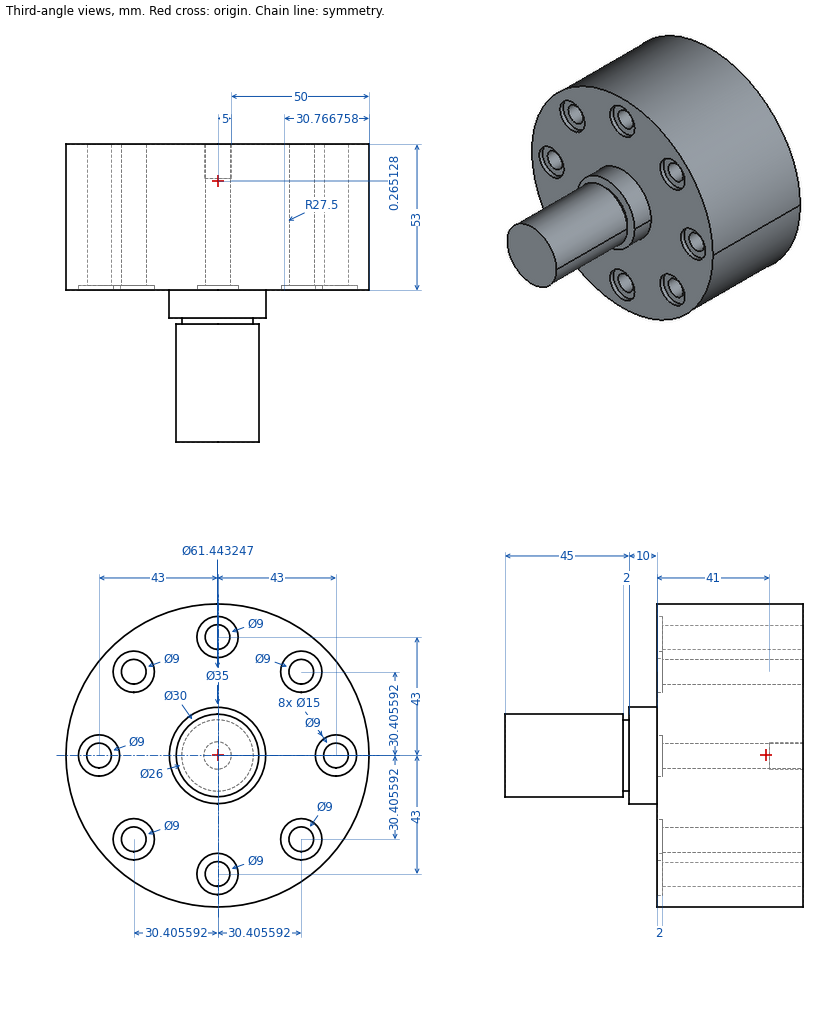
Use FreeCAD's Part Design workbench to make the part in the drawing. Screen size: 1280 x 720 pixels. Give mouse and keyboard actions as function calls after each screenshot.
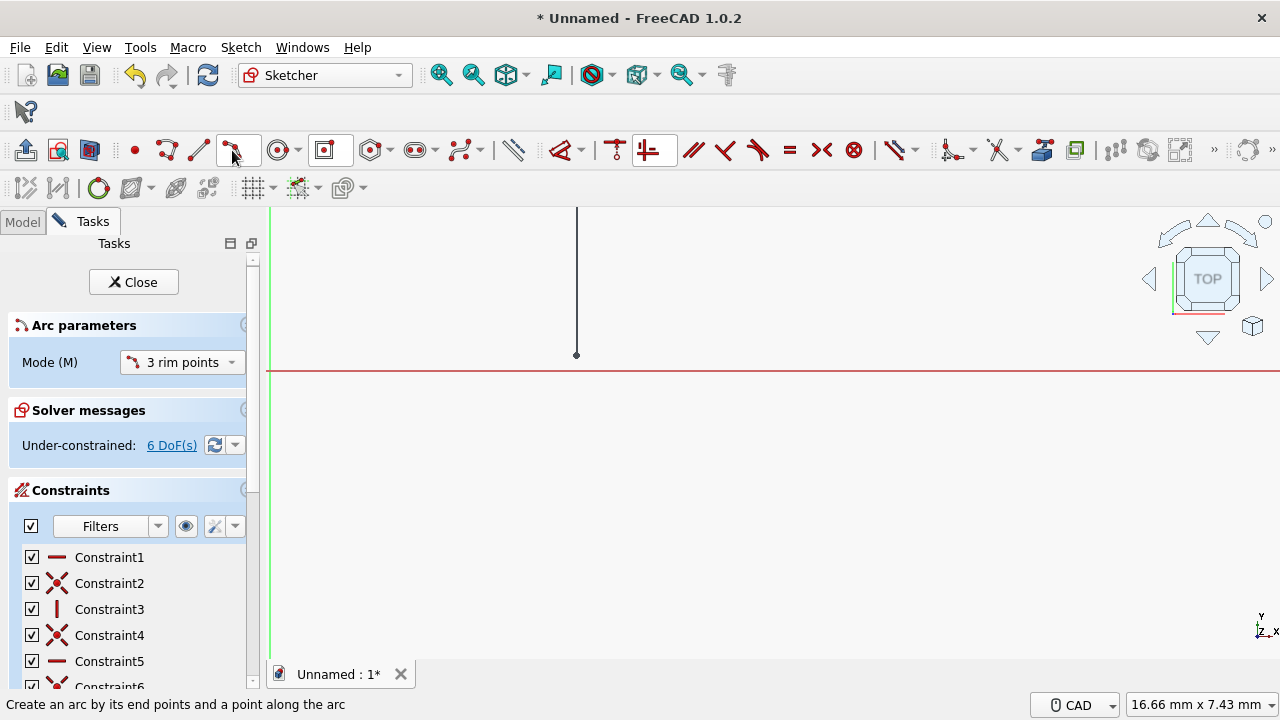
click(577, 356)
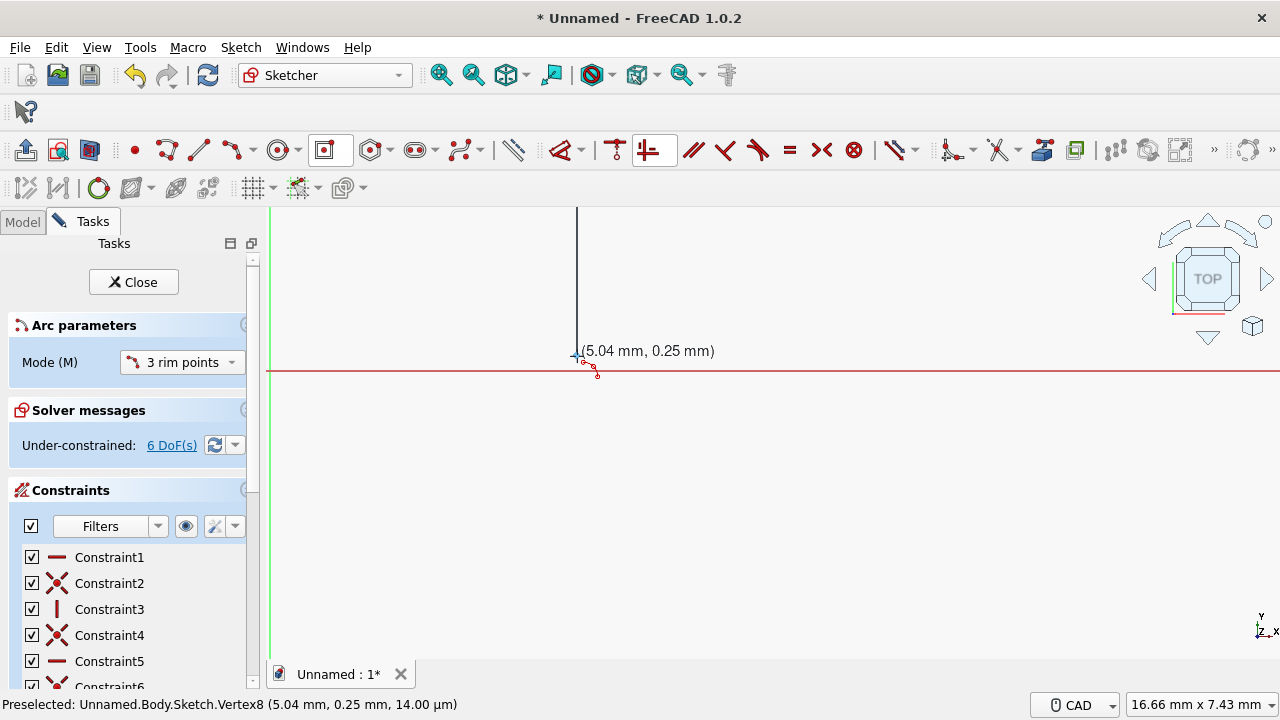
scroll(581, 359, down, 12)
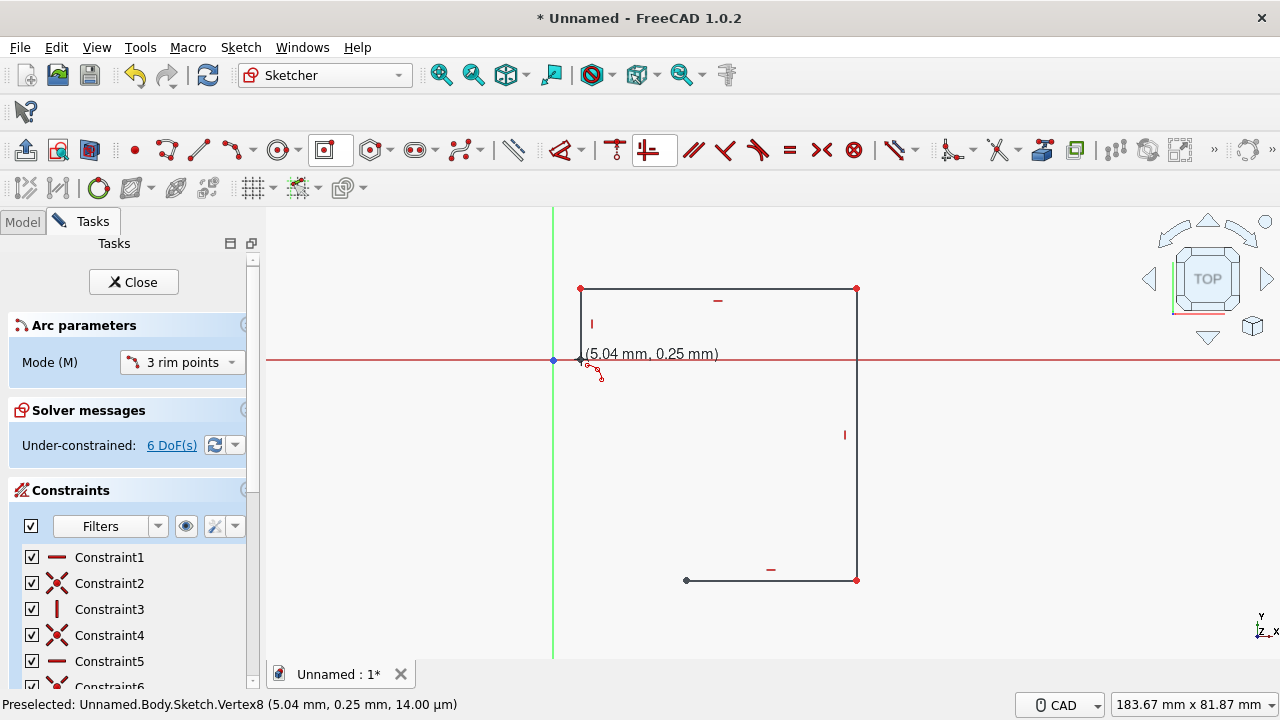
click(687, 581)
click(690, 443)
key(Escape)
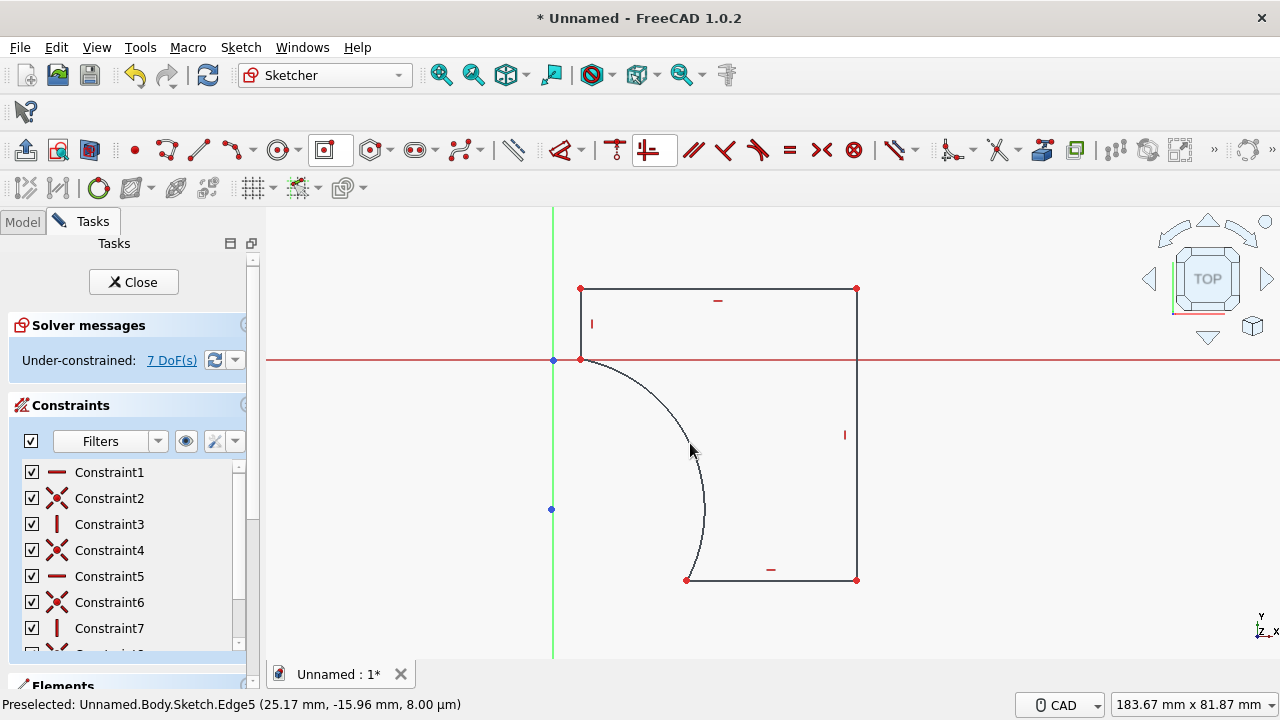
click(551, 509)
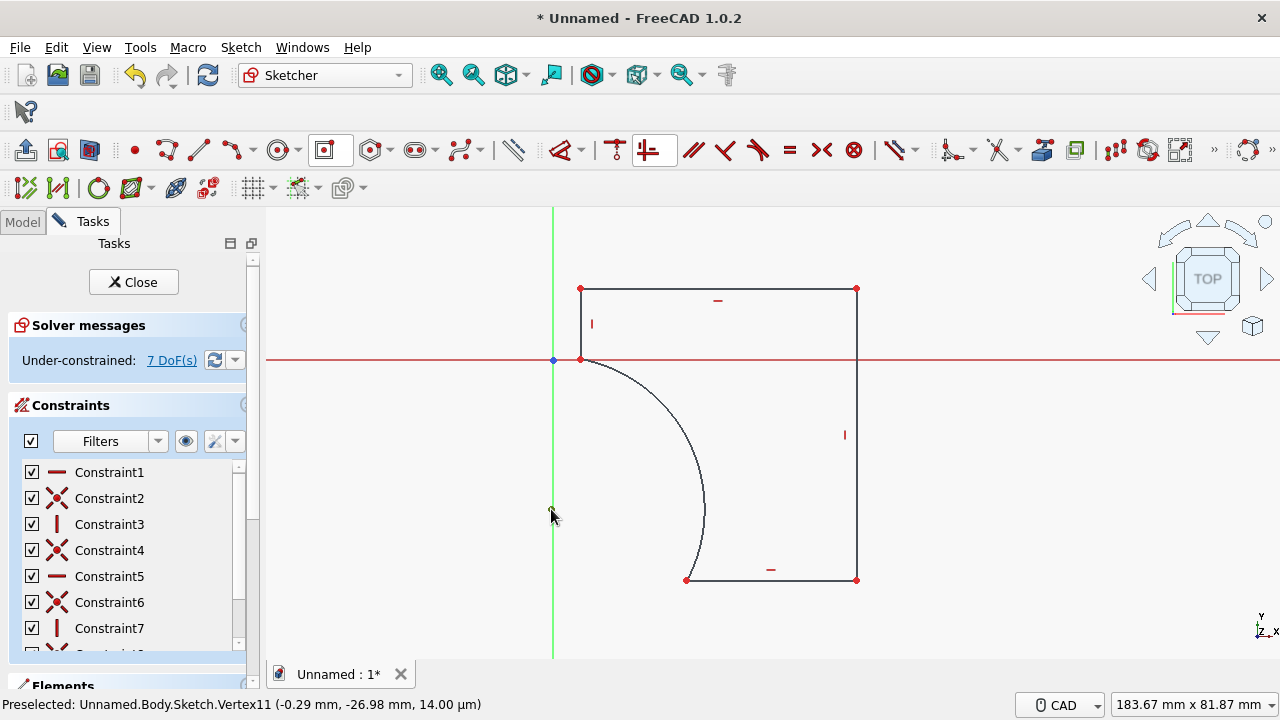
click(553, 603)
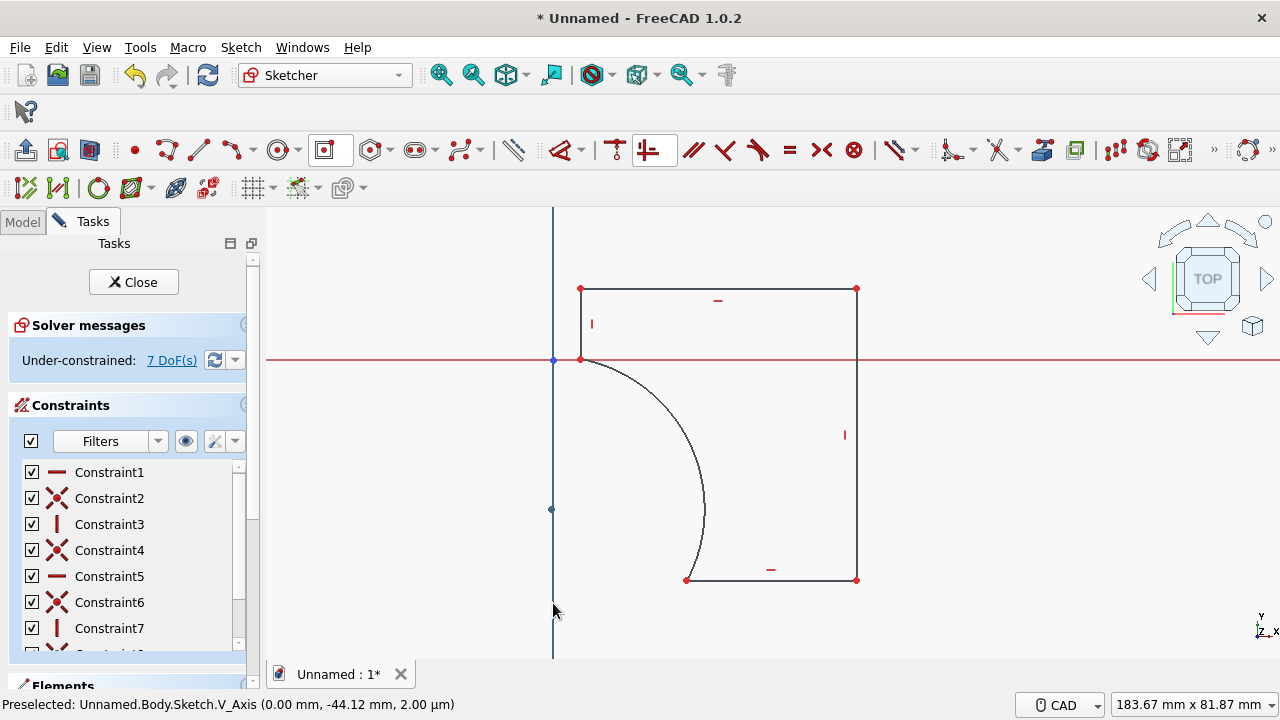
click(616, 150)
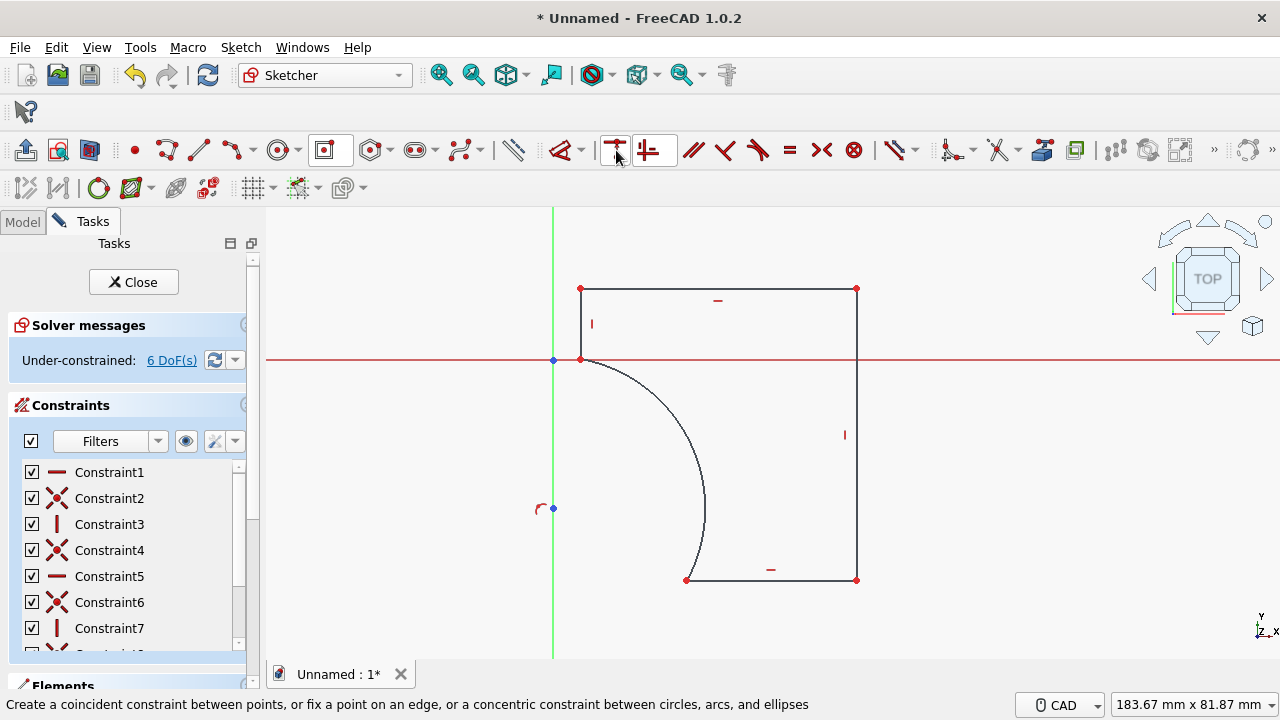
click(705, 498)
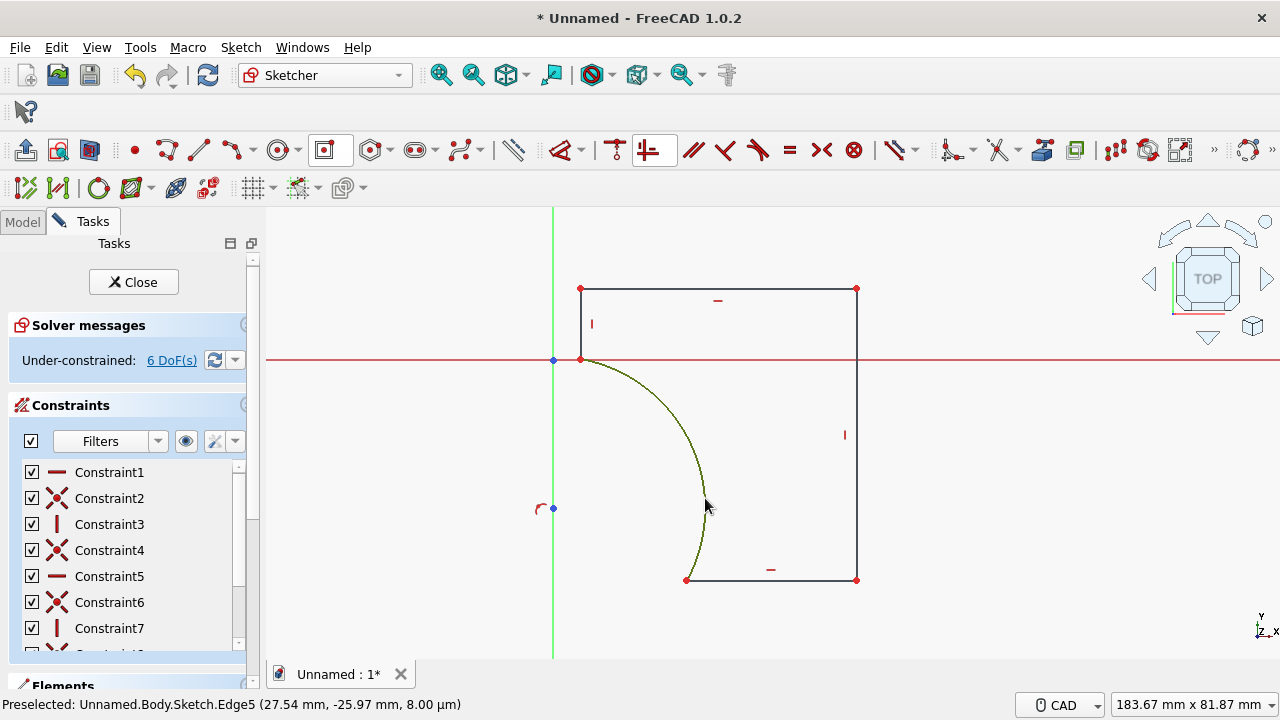
click(584, 150)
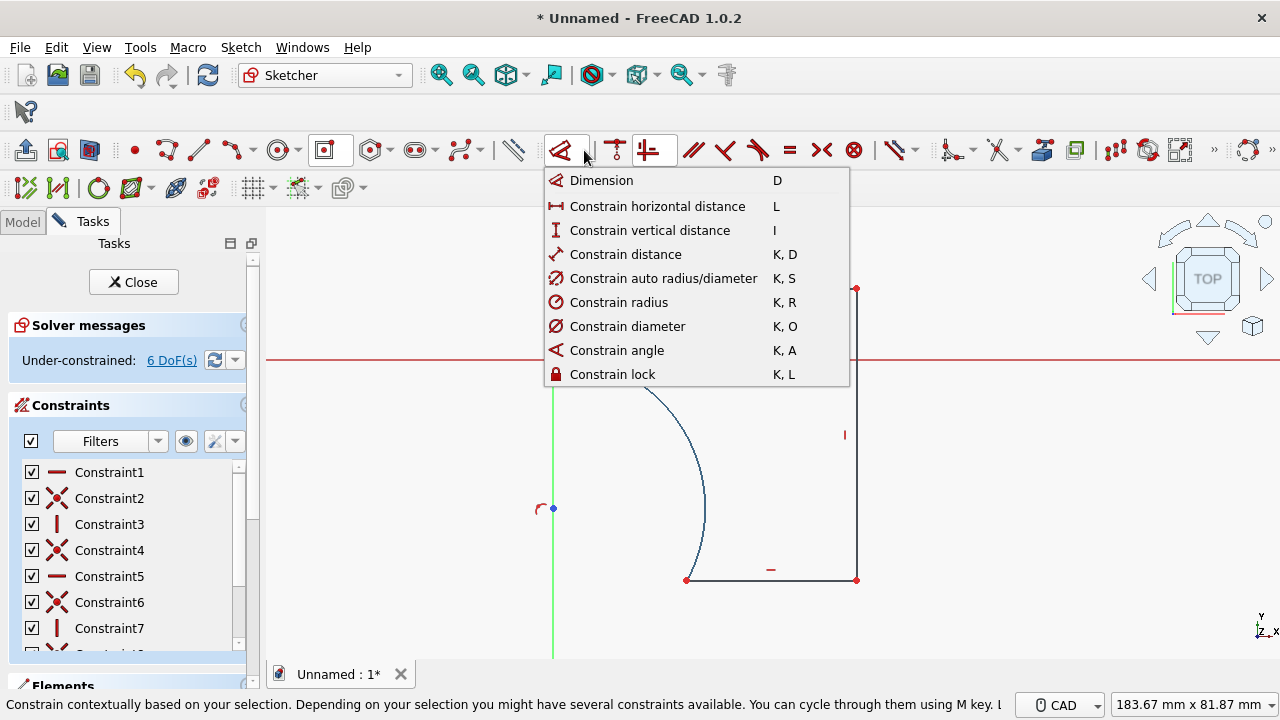
click(697, 302)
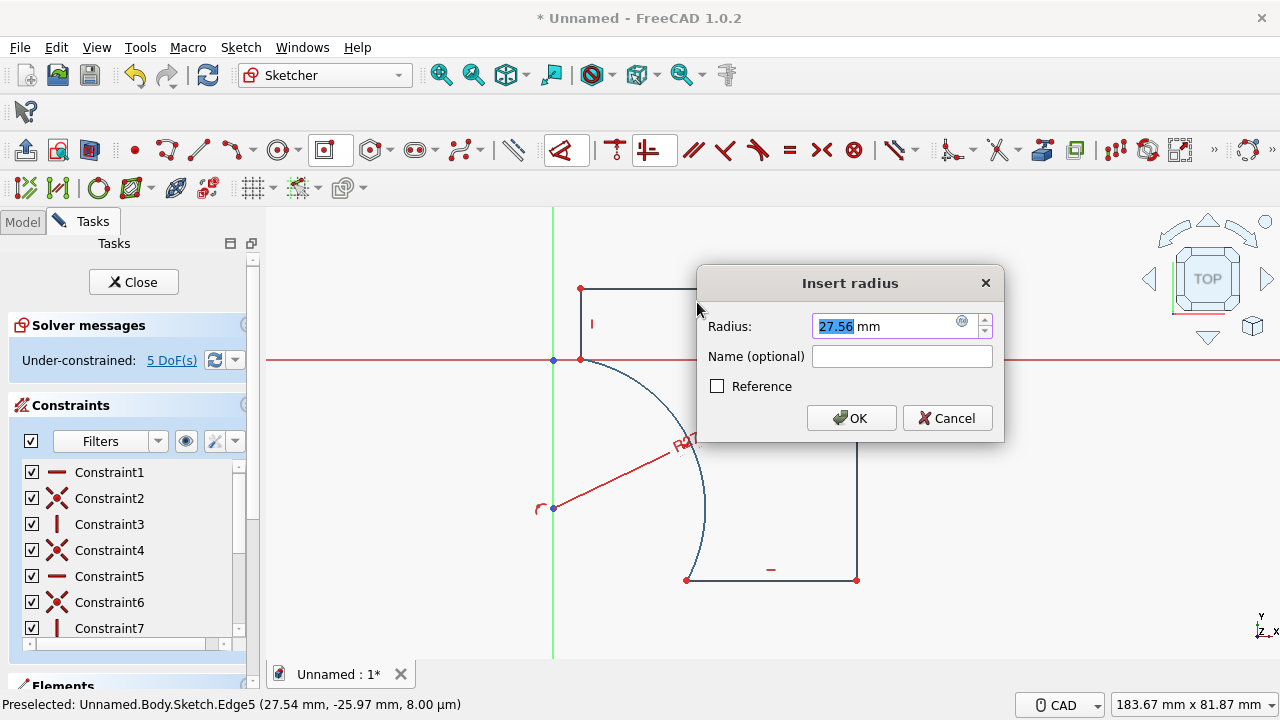
text(27.5)
key(Return)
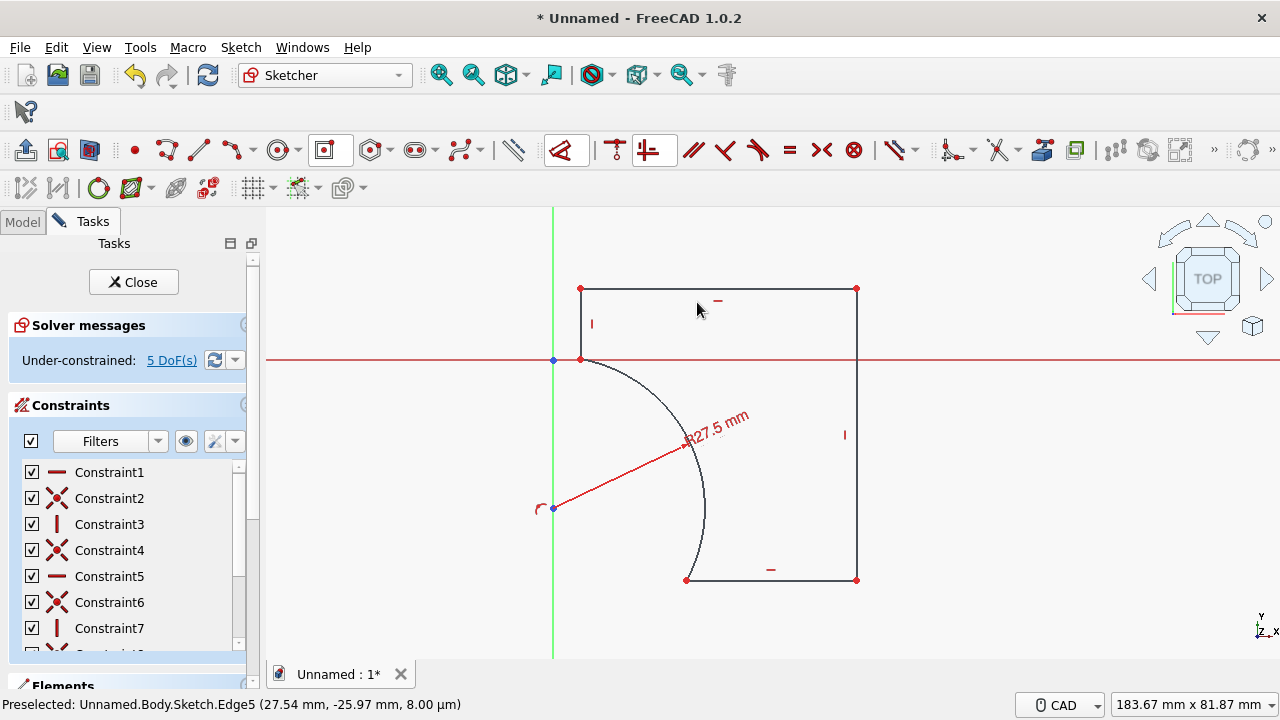
click(857, 493)